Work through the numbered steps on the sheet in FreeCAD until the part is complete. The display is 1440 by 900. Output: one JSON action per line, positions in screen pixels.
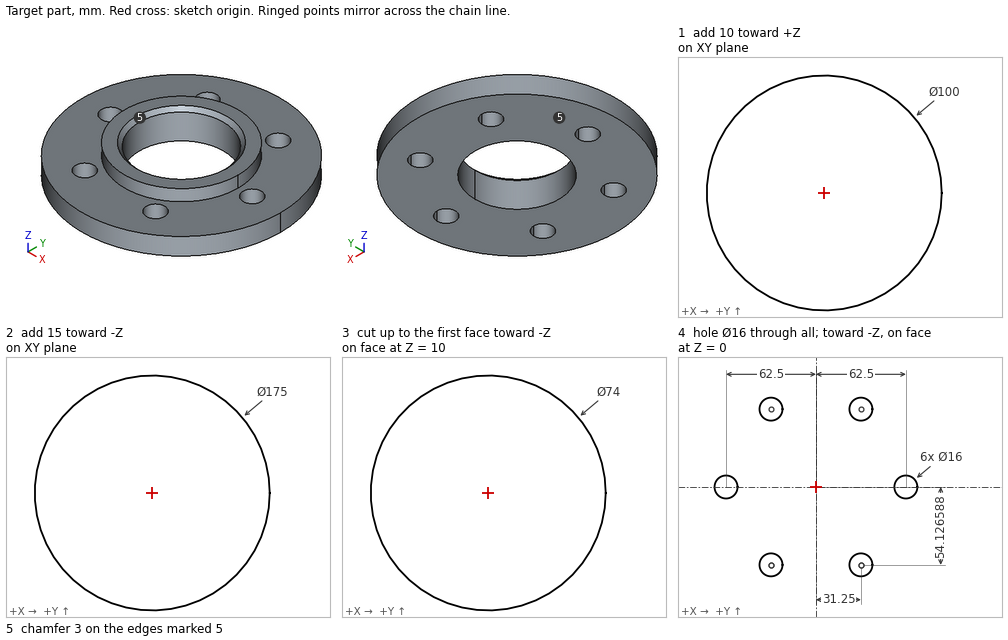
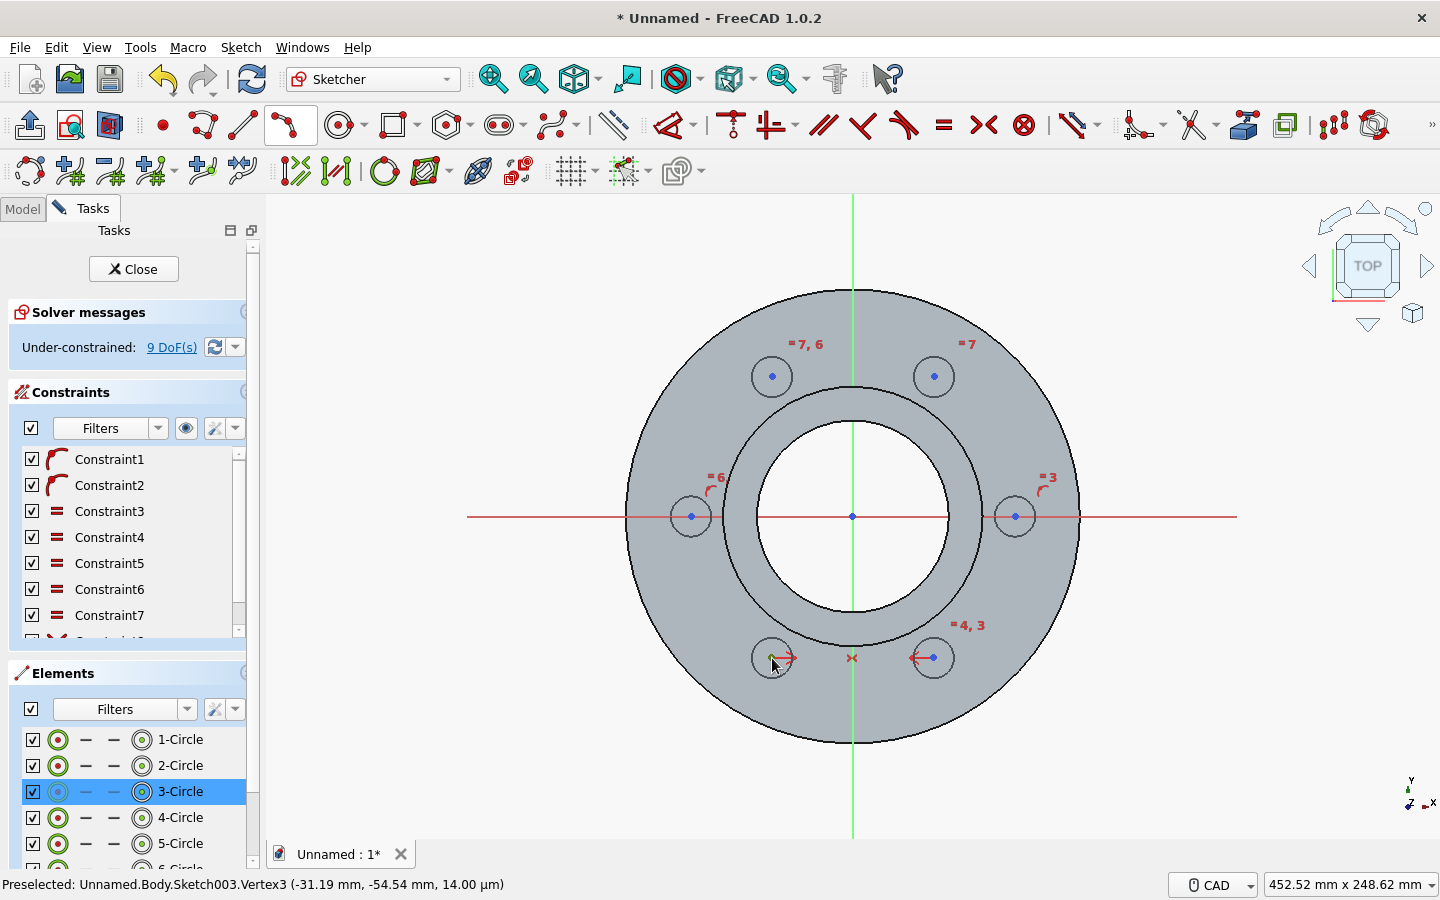
{"action": "left_click", "coordinate": [772, 377]}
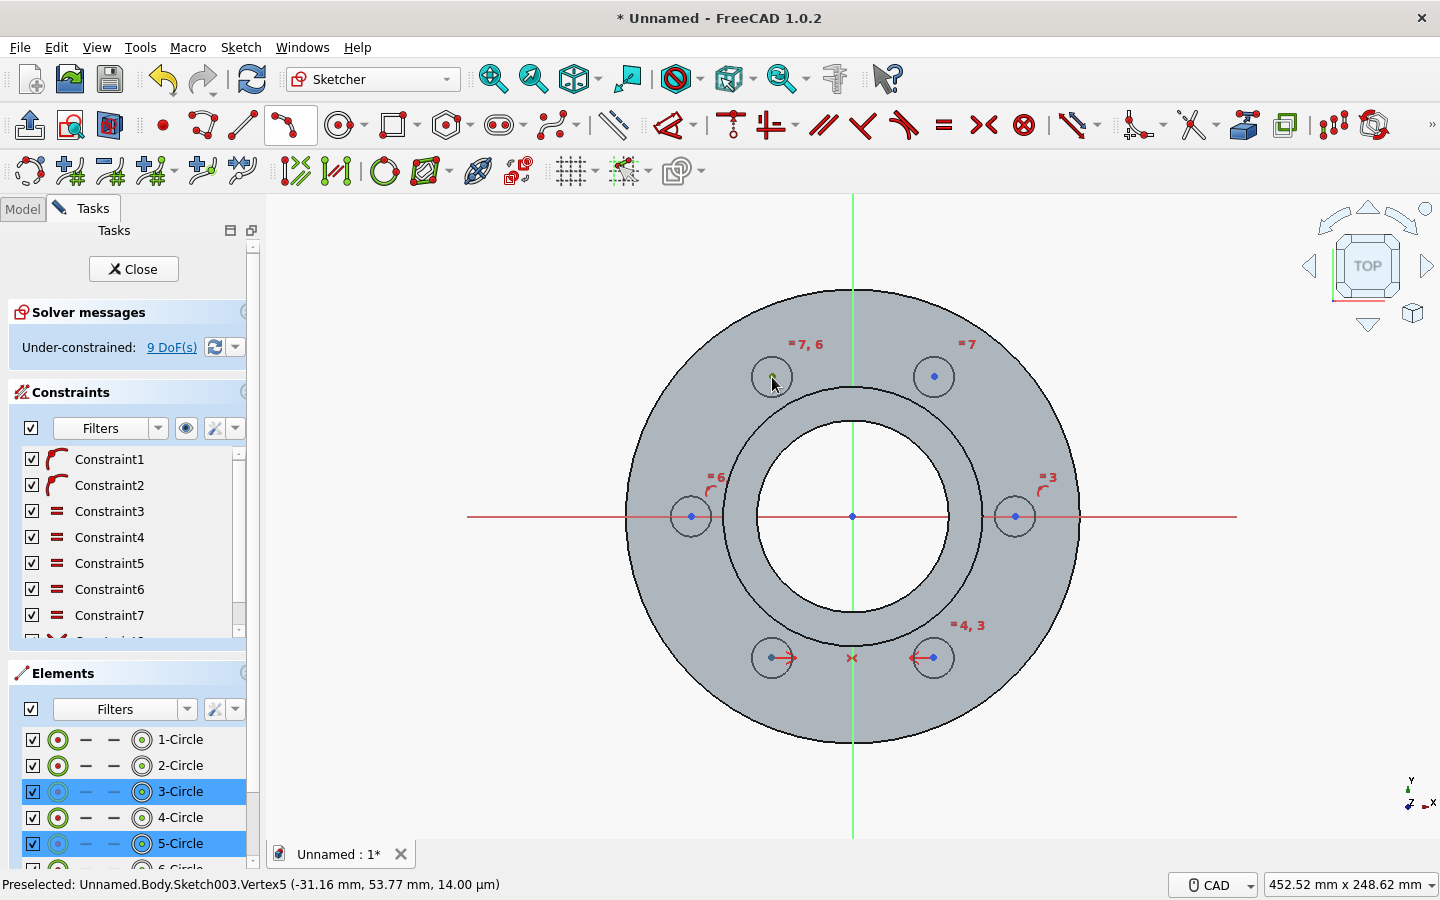
{"action": "left_click", "coordinate": [504, 516]}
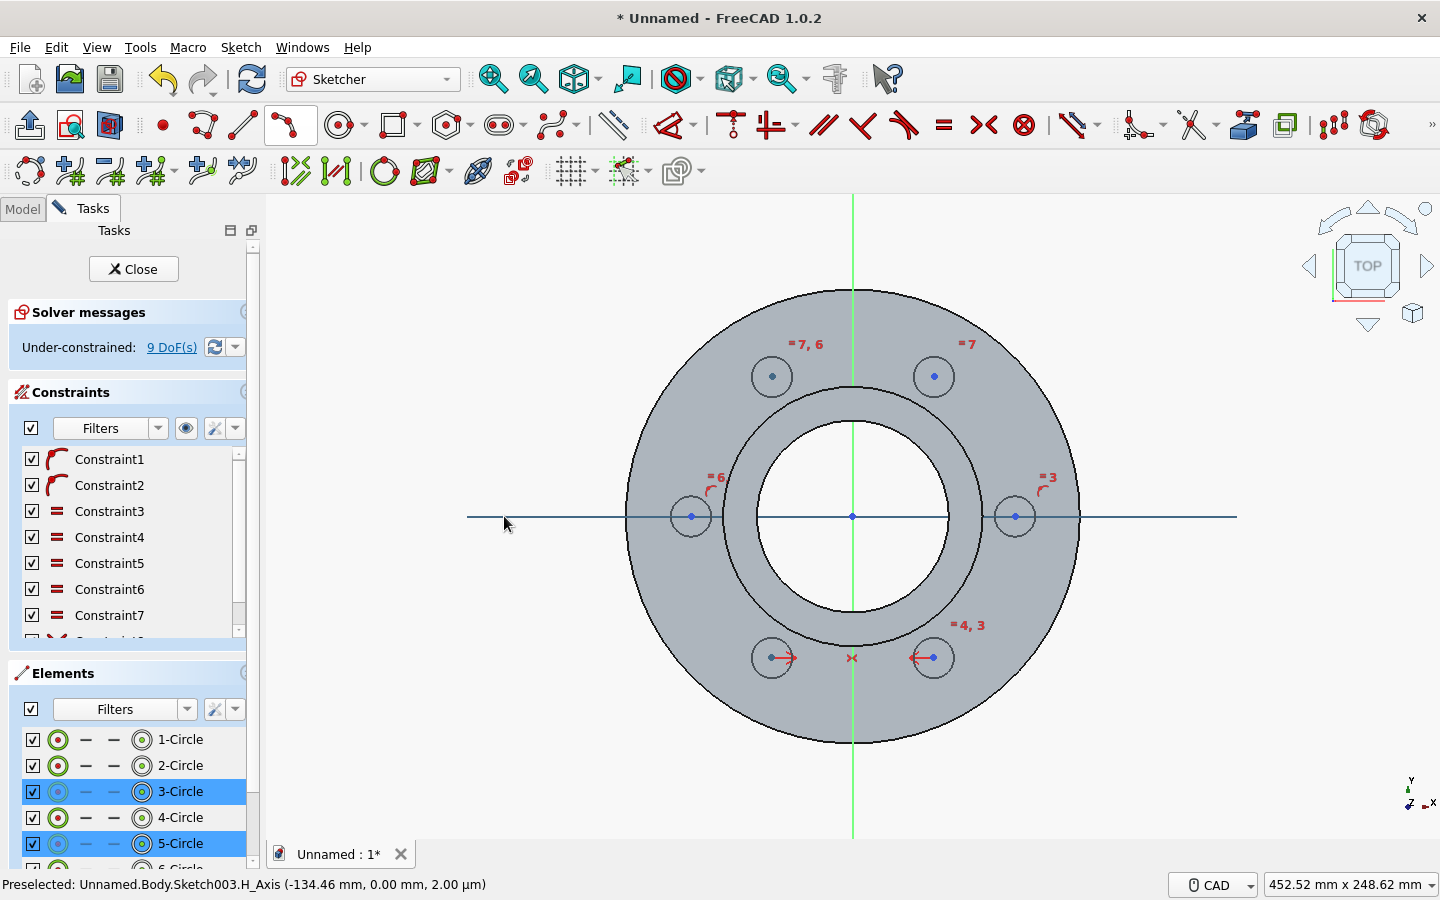
{"action": "key", "text": "s"}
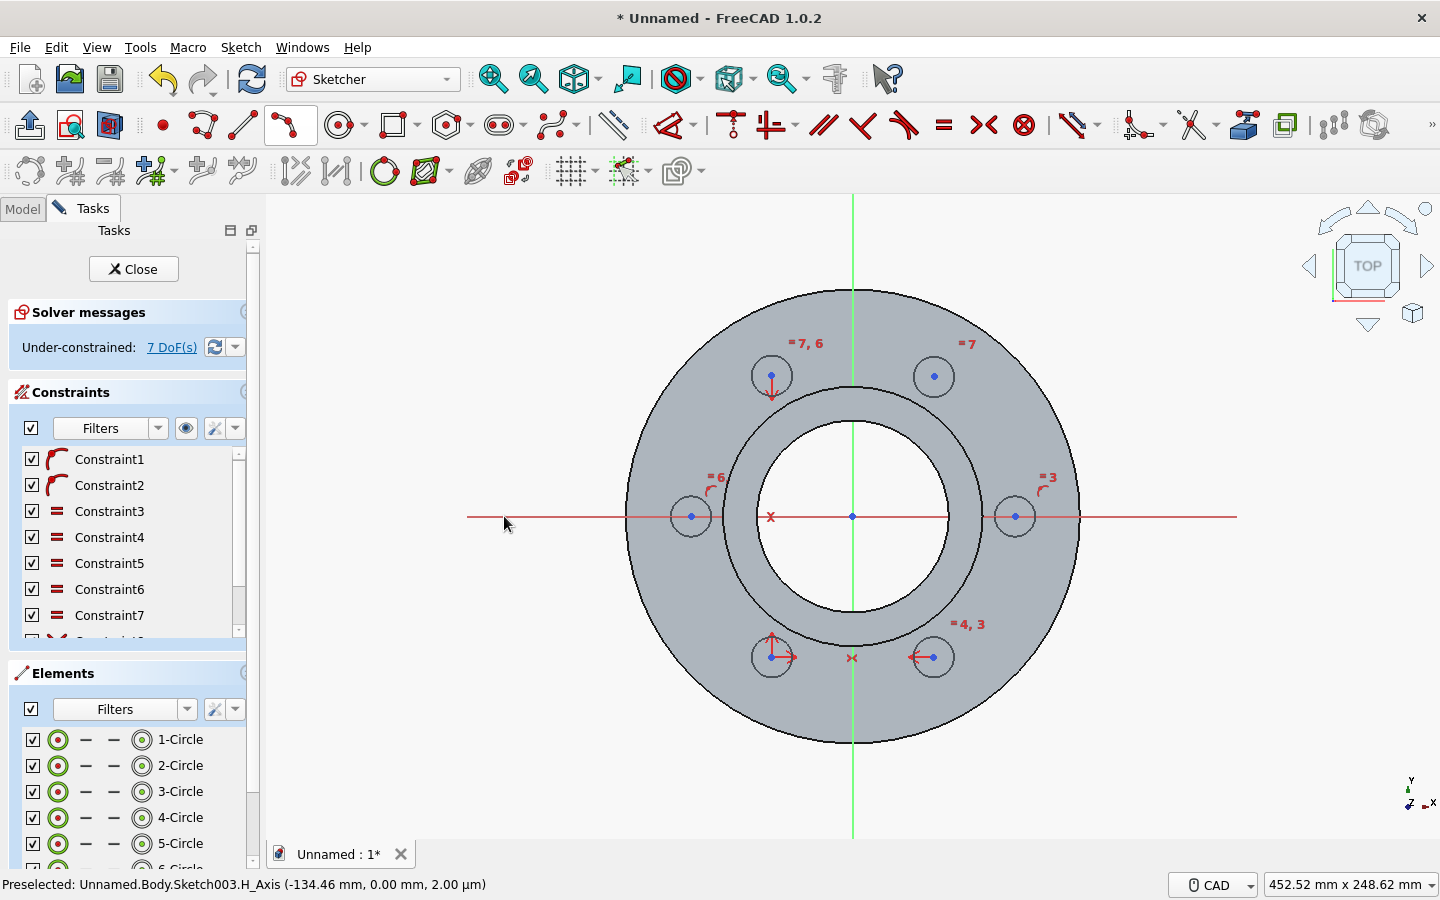
{"action": "left_click", "coordinate": [934, 657]}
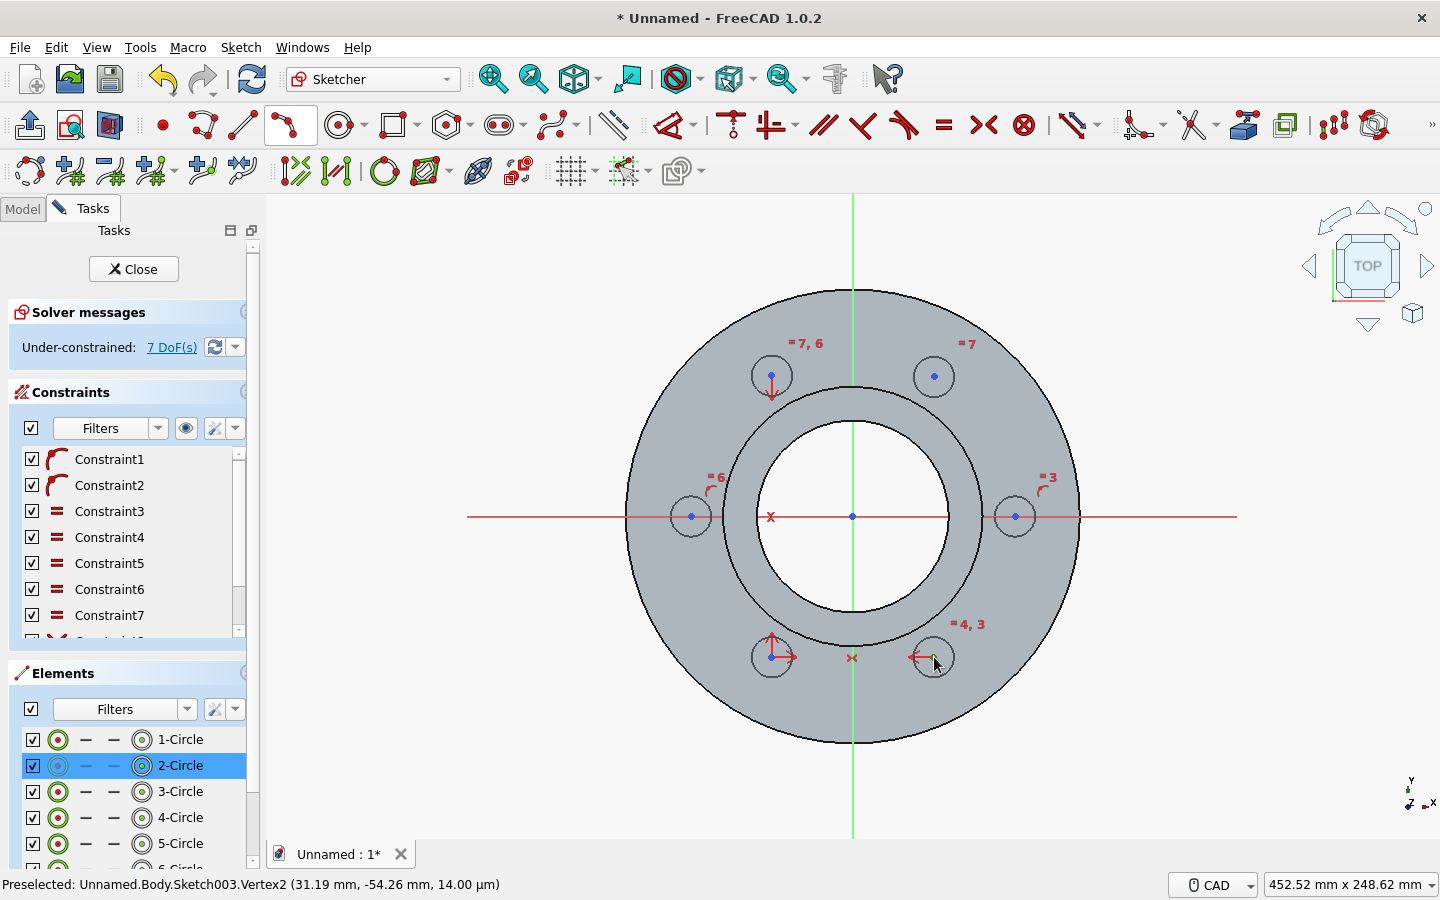
{"action": "left_click", "coordinate": [934, 377]}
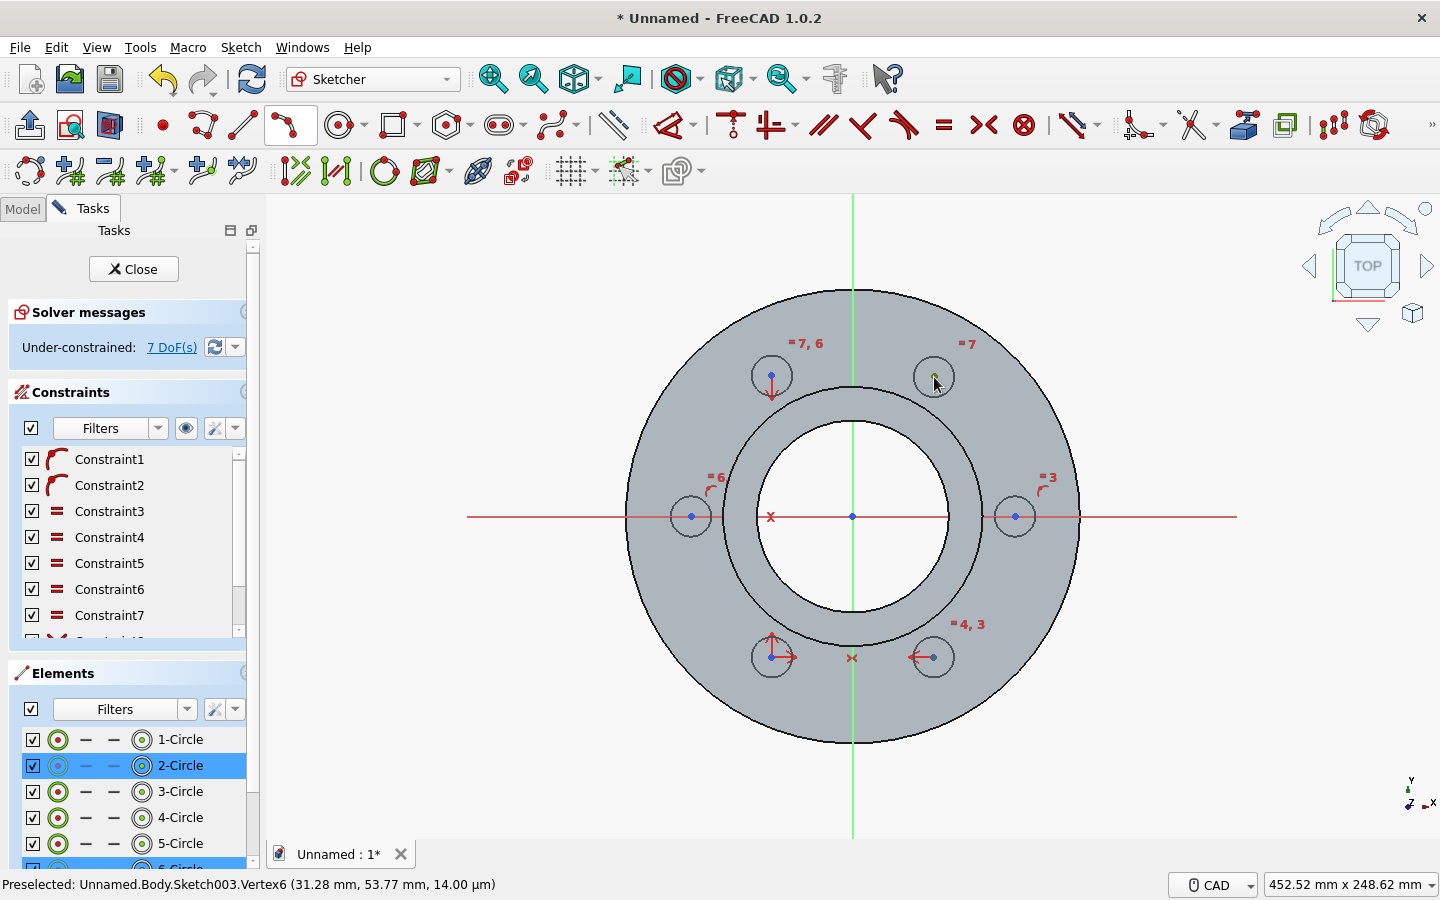
{"action": "left_click", "coordinate": [504, 516]}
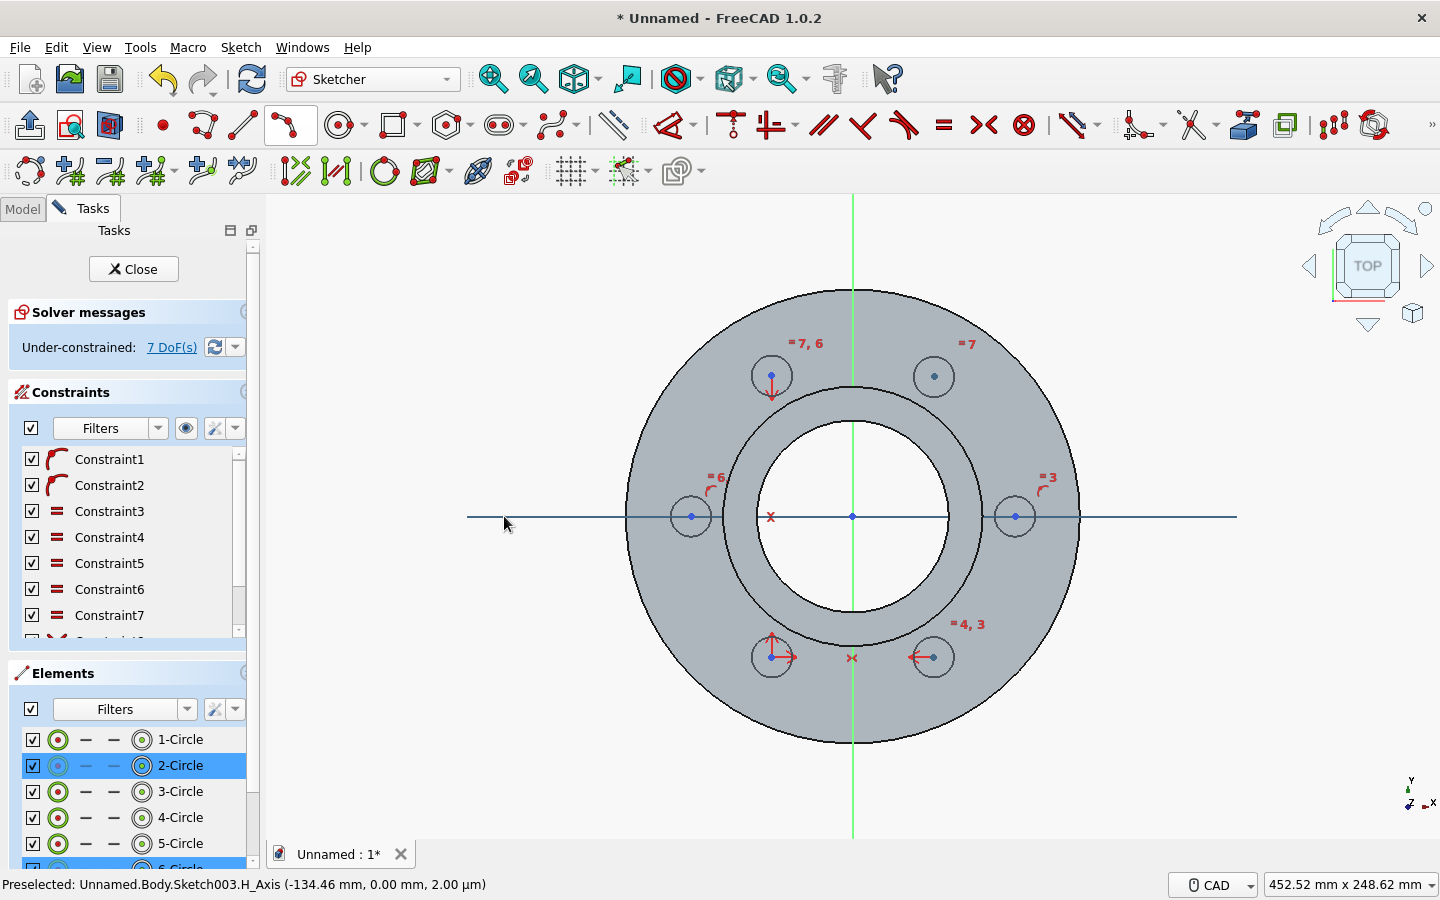
{"action": "left_click", "coordinate": [984, 126]}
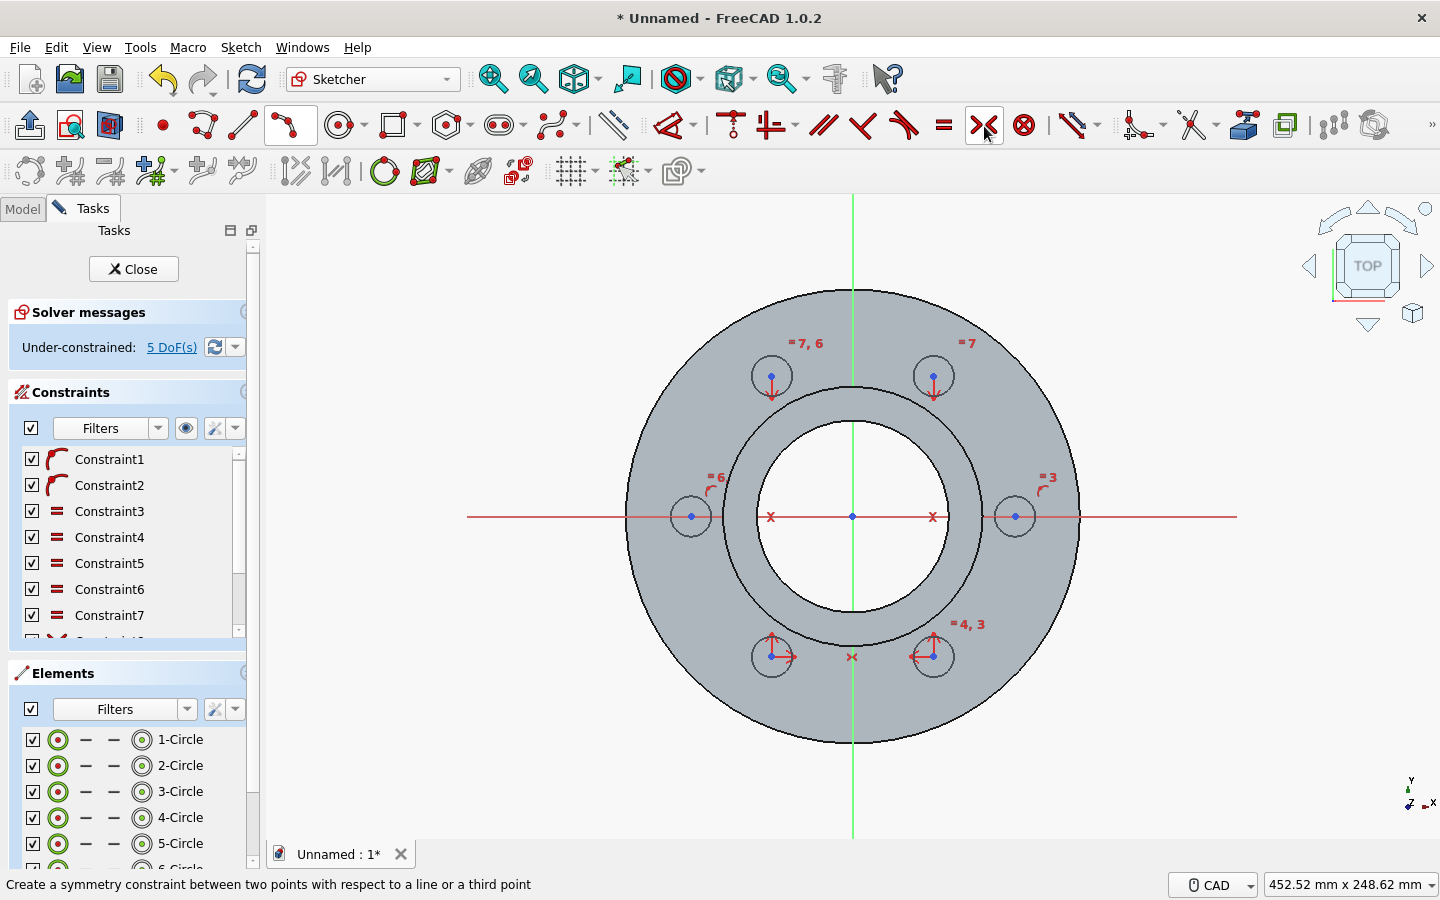
{"action": "left_click", "coordinate": [668, 126]}